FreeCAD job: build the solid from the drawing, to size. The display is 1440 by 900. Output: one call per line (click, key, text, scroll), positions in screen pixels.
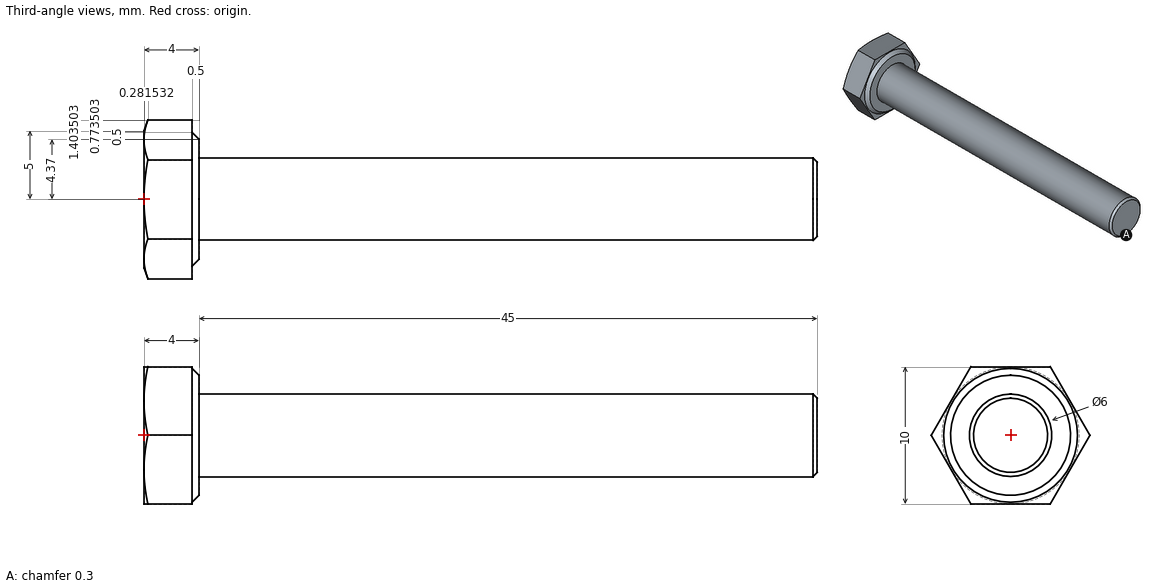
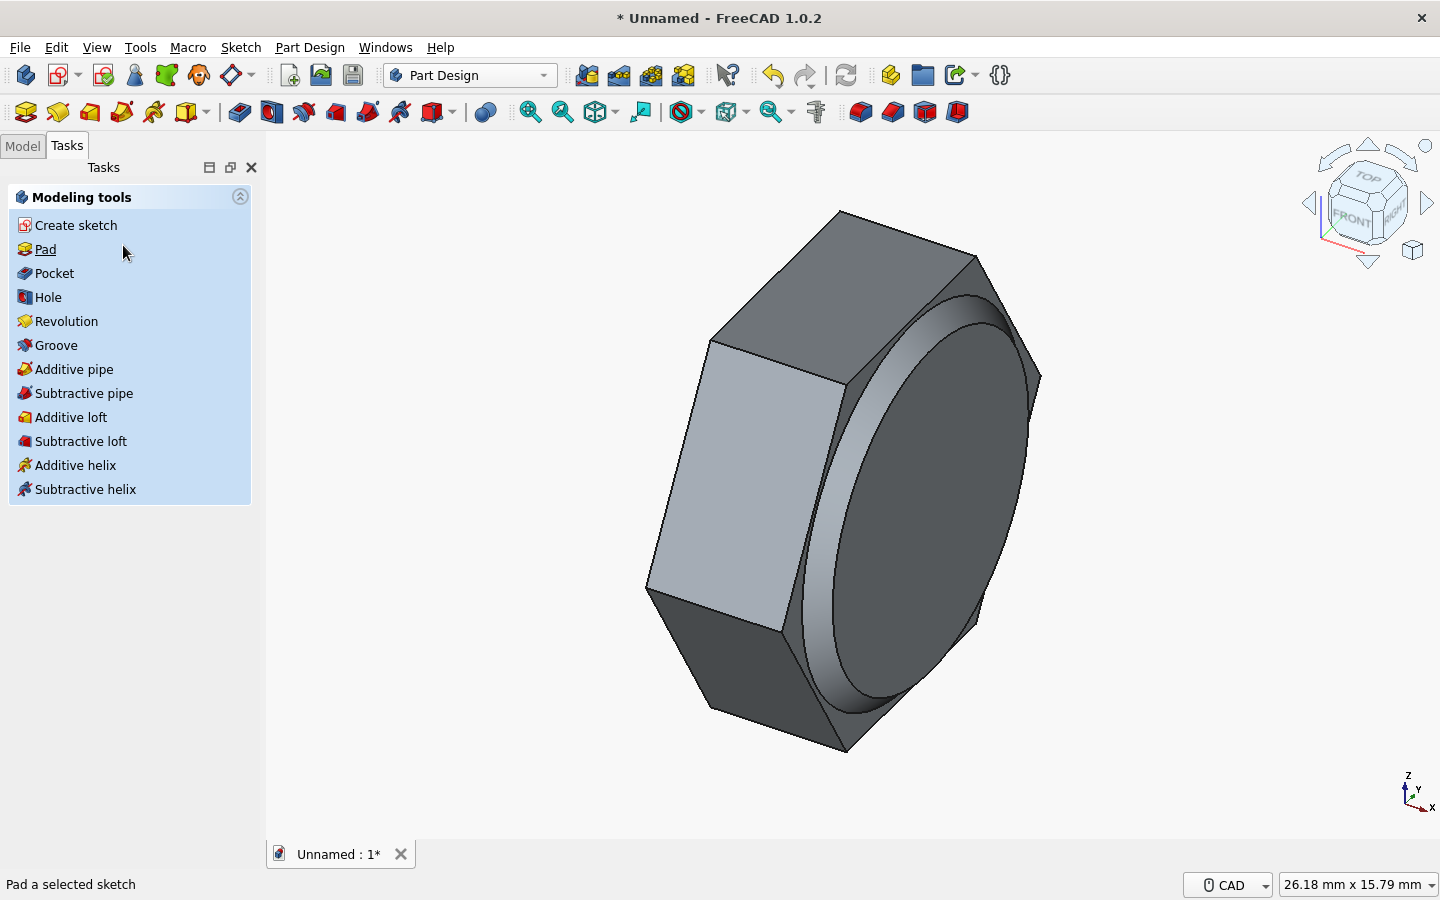
click(304, 112)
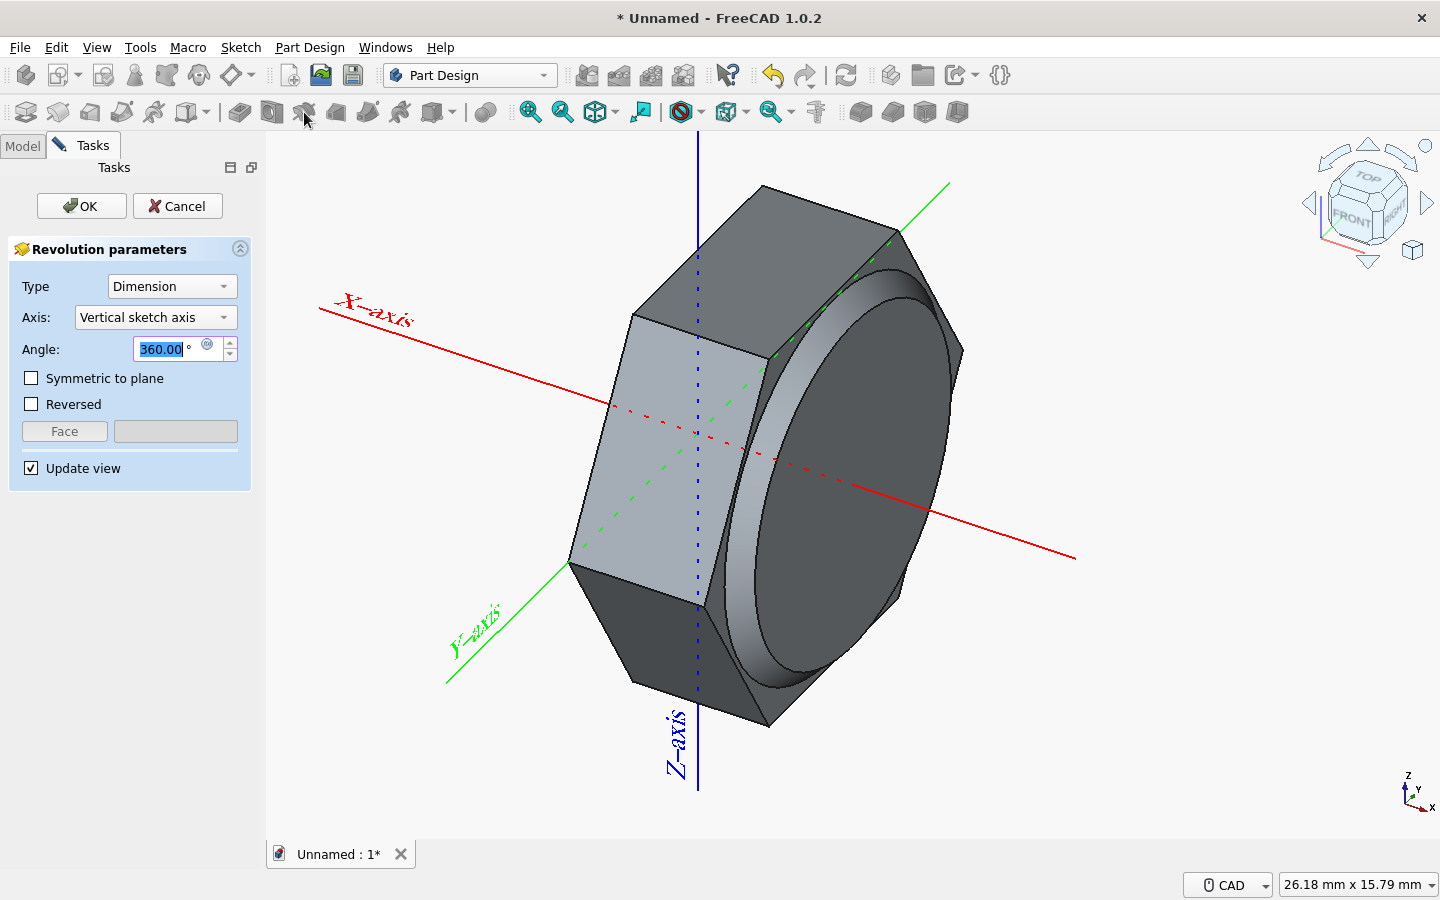
click(156, 318)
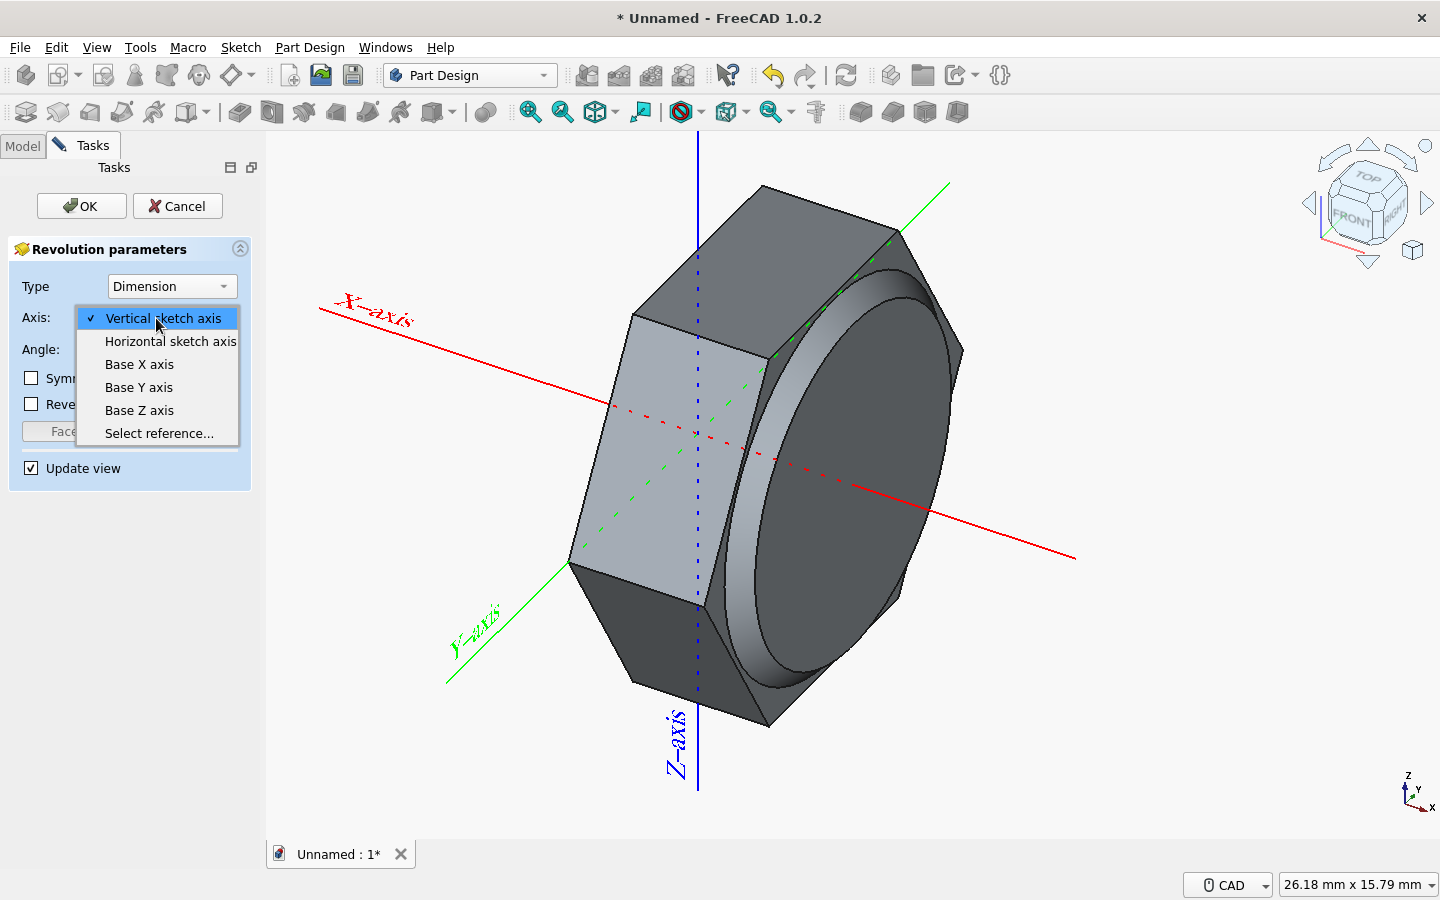
click(156, 342)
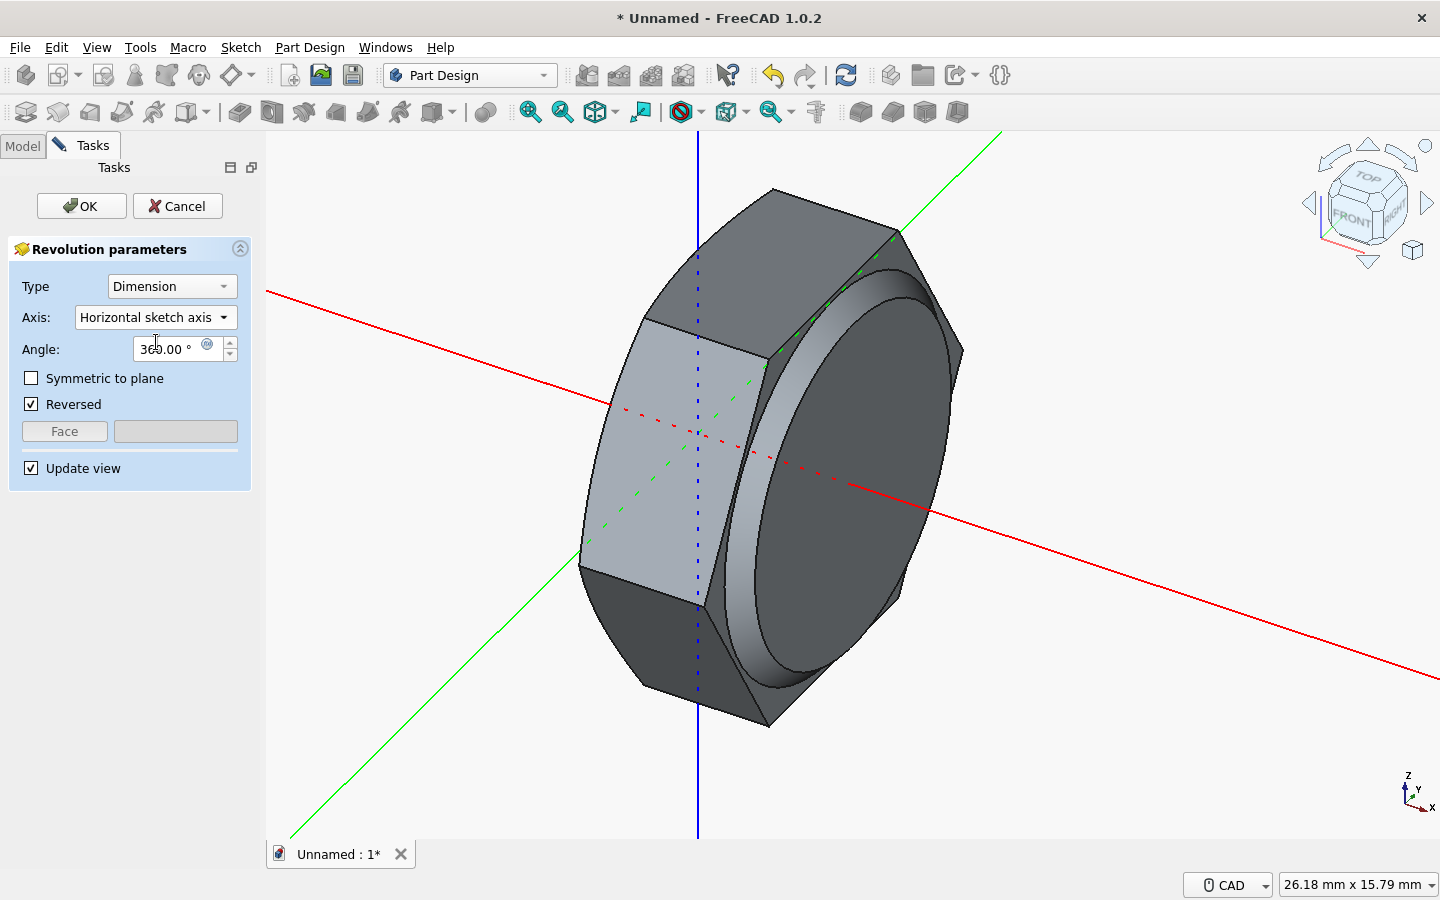
click(82, 206)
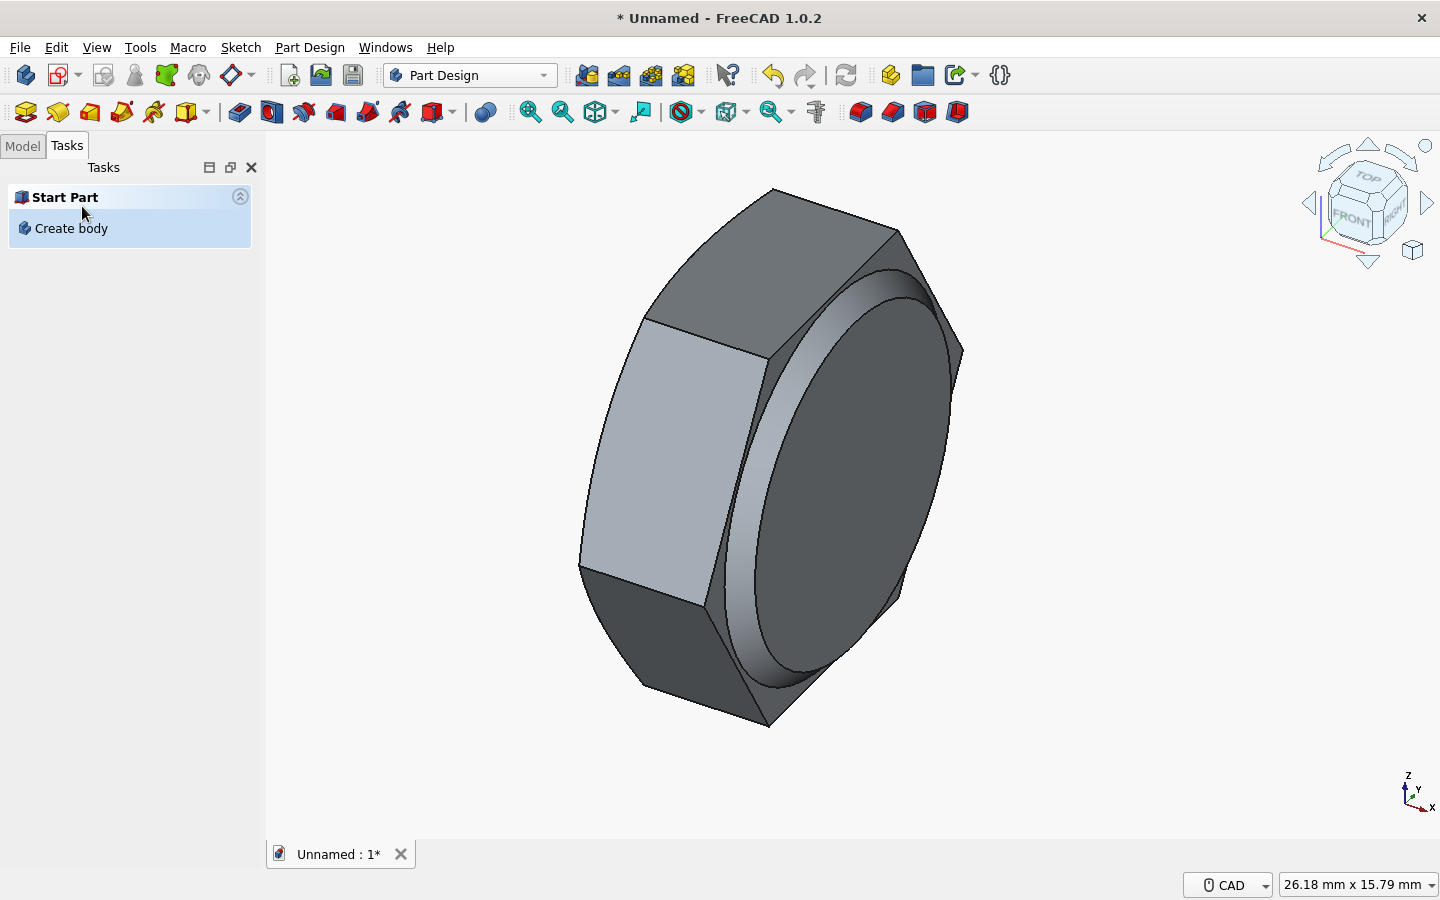
click(532, 112)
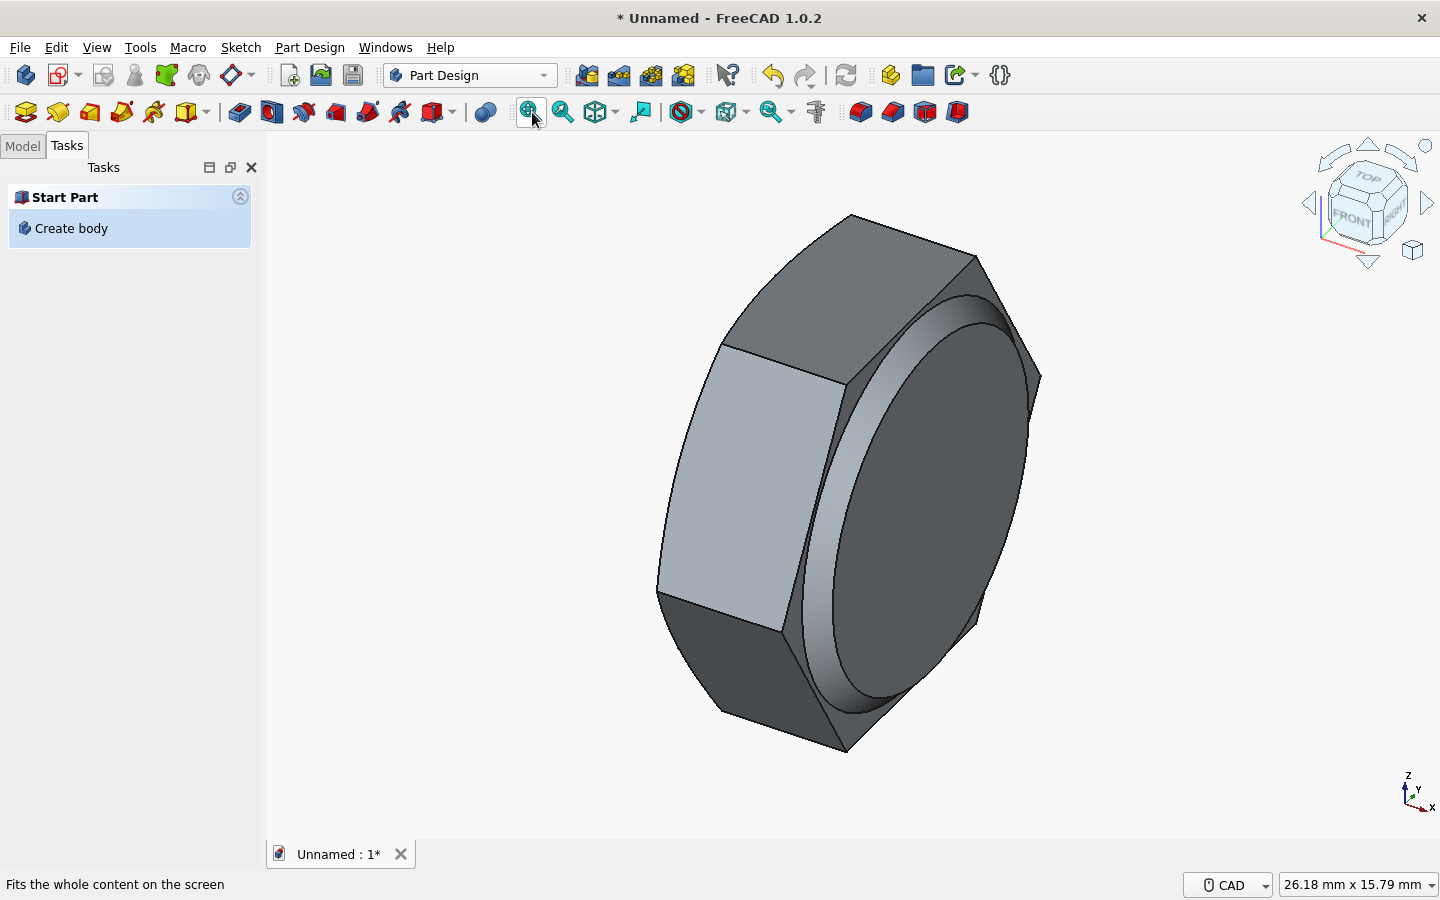
click(931, 510)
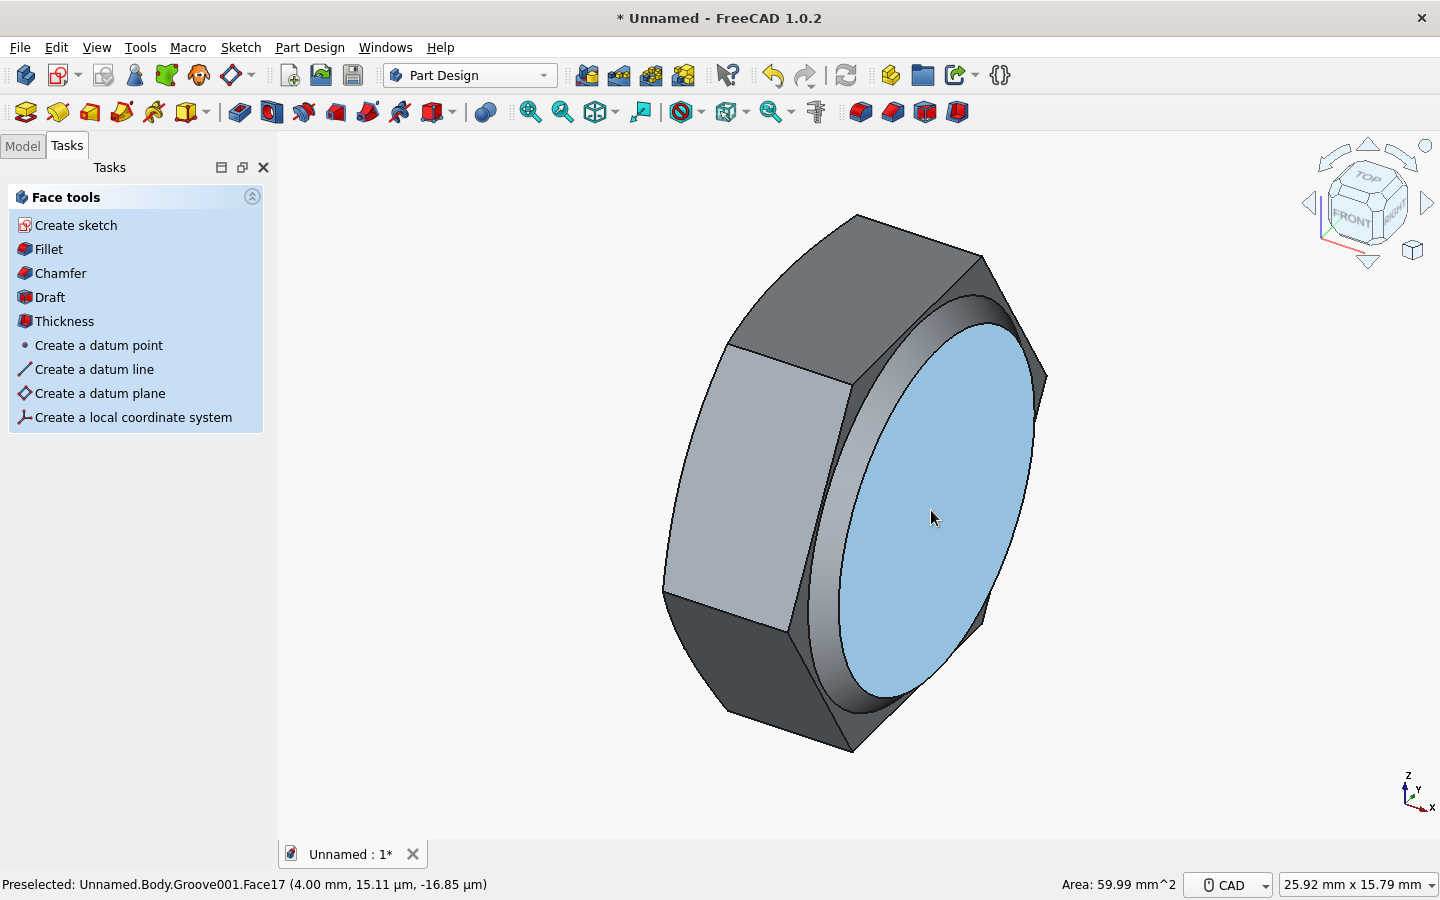
click(58, 76)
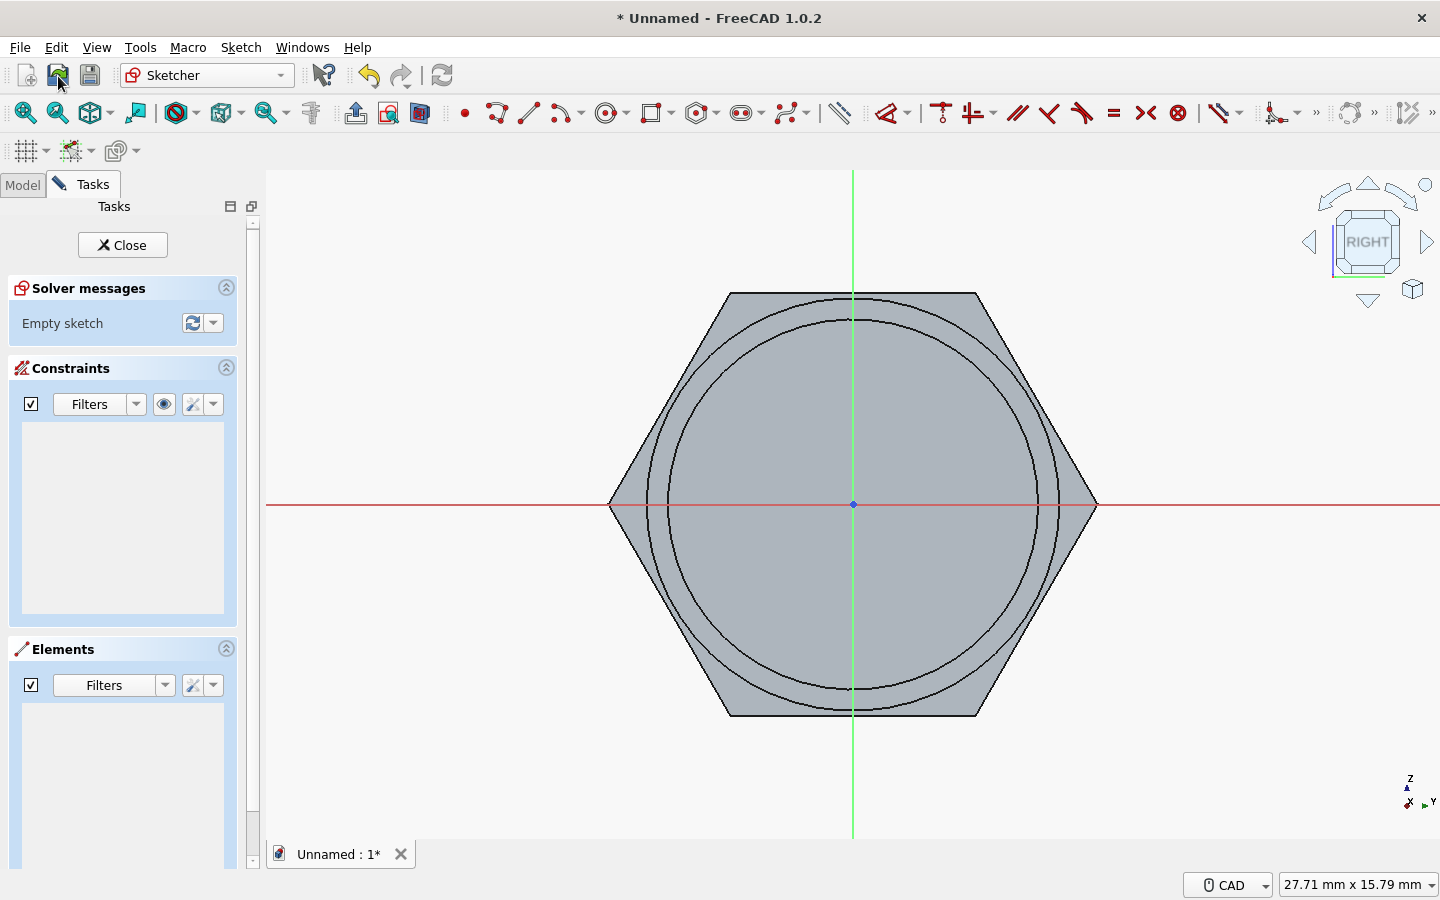
scroll(936, 504, up, 3)